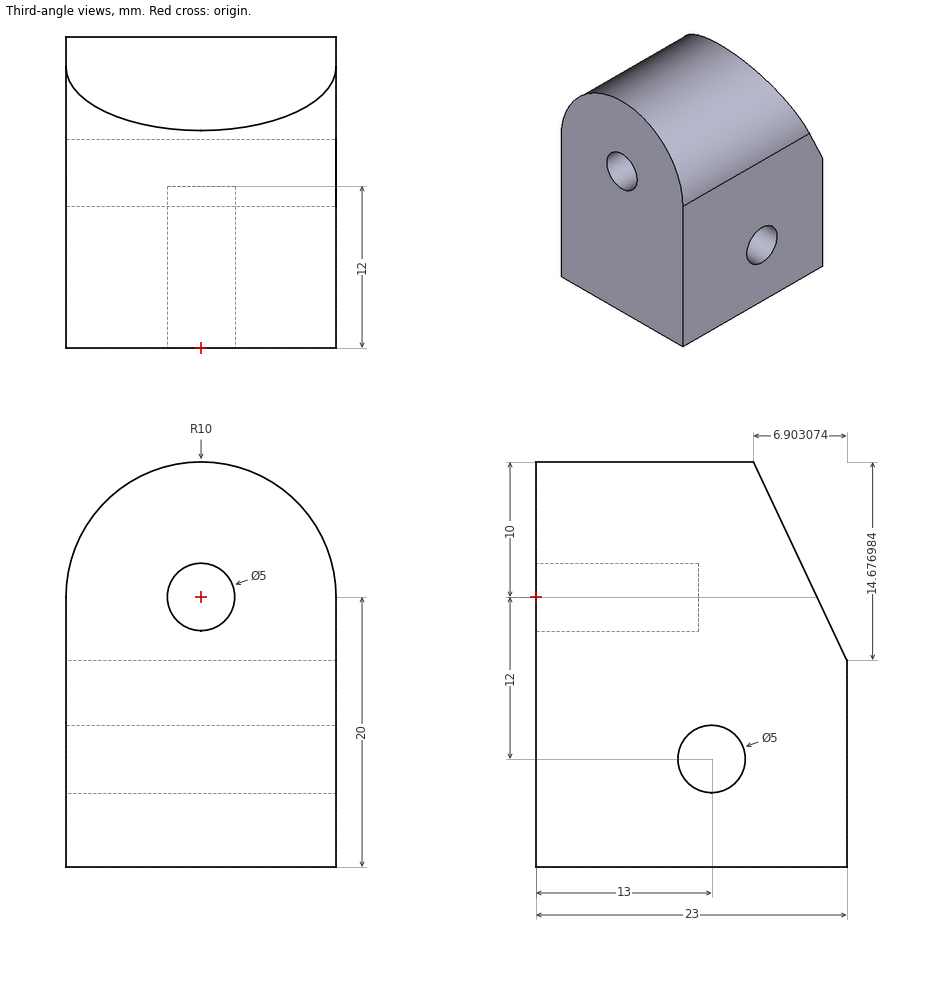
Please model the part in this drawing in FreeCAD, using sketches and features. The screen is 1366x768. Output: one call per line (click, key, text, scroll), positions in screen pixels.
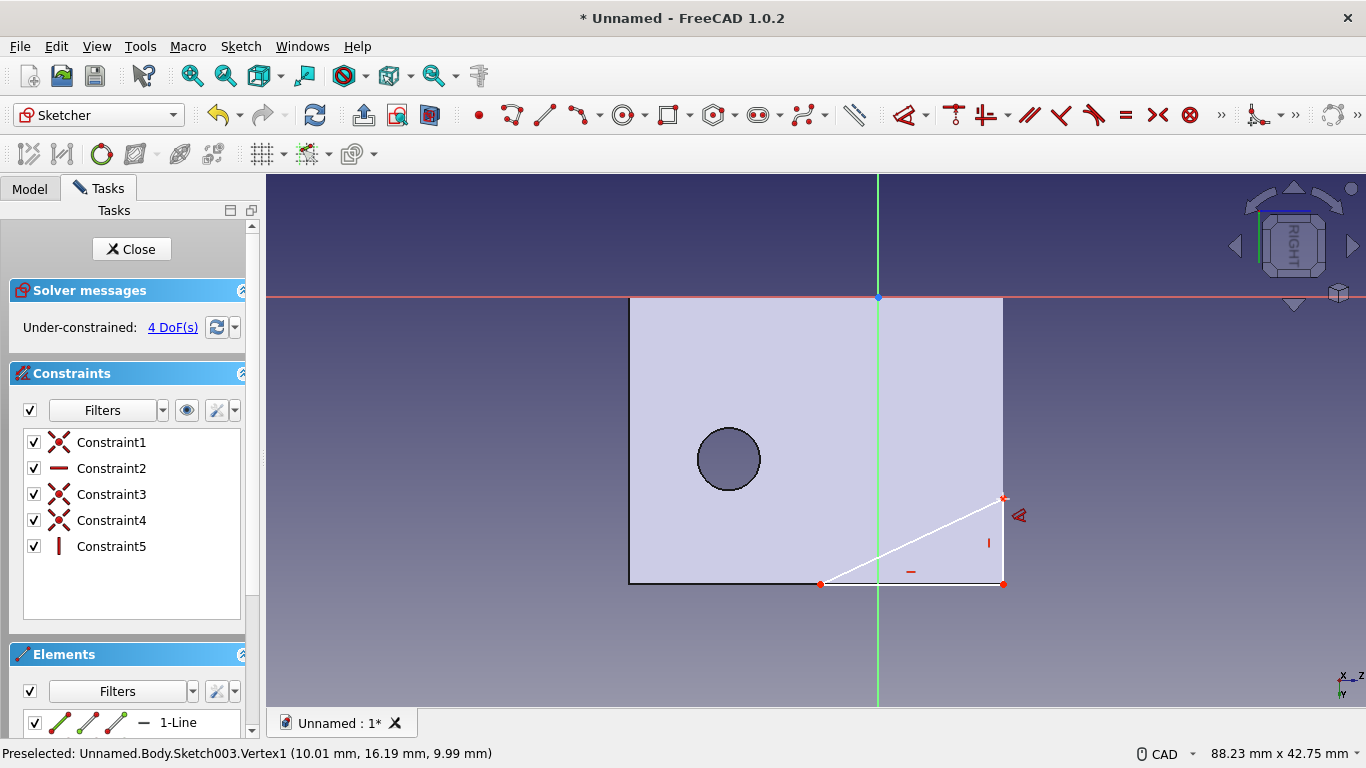
click(1003, 499)
click(941, 263)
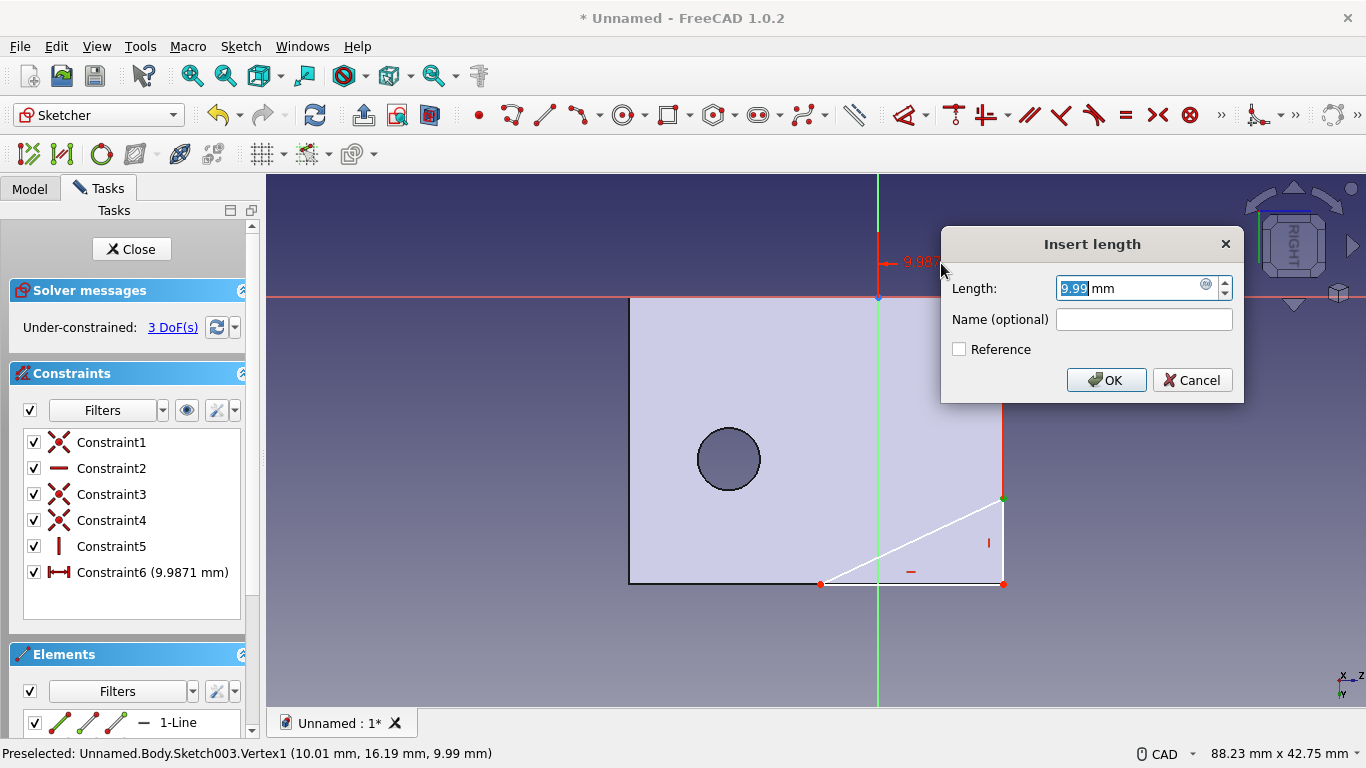
text(10)
key(Return)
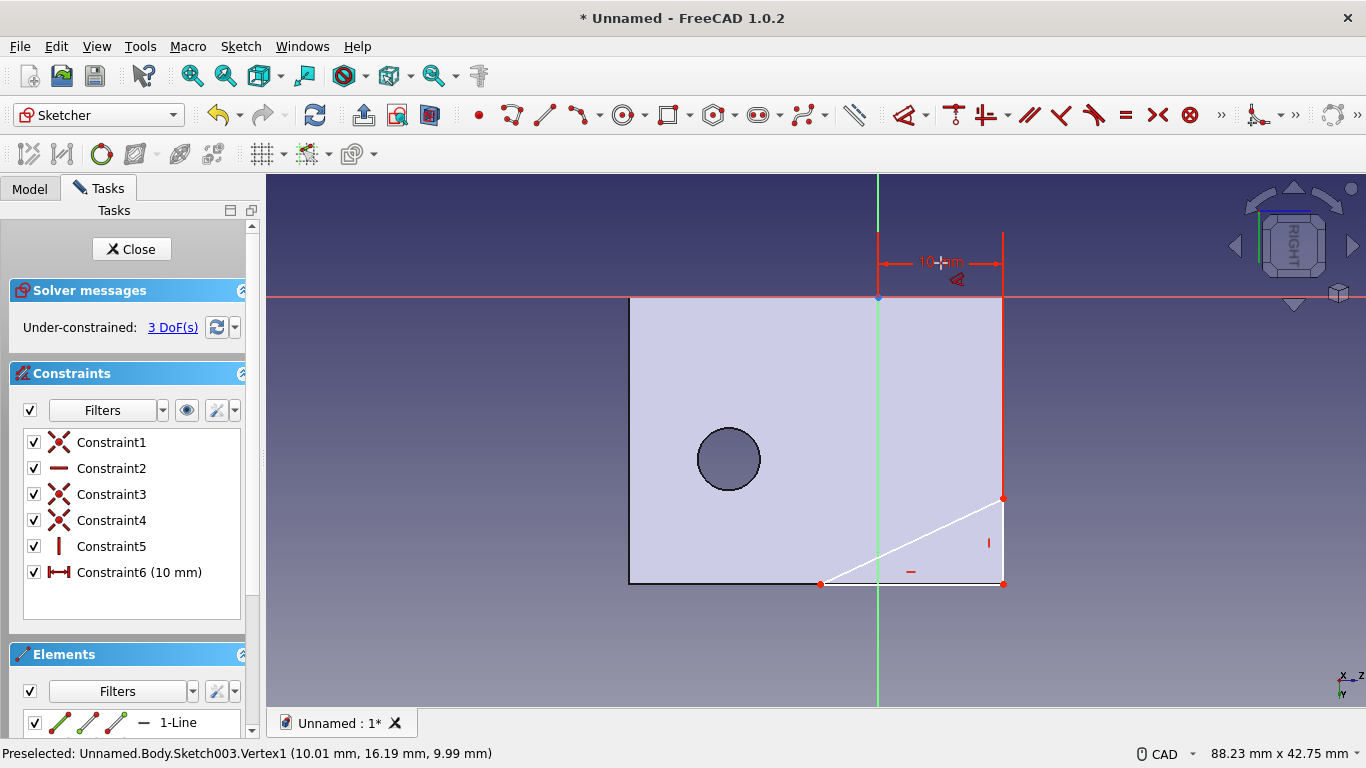
click(820, 585)
click(786, 441)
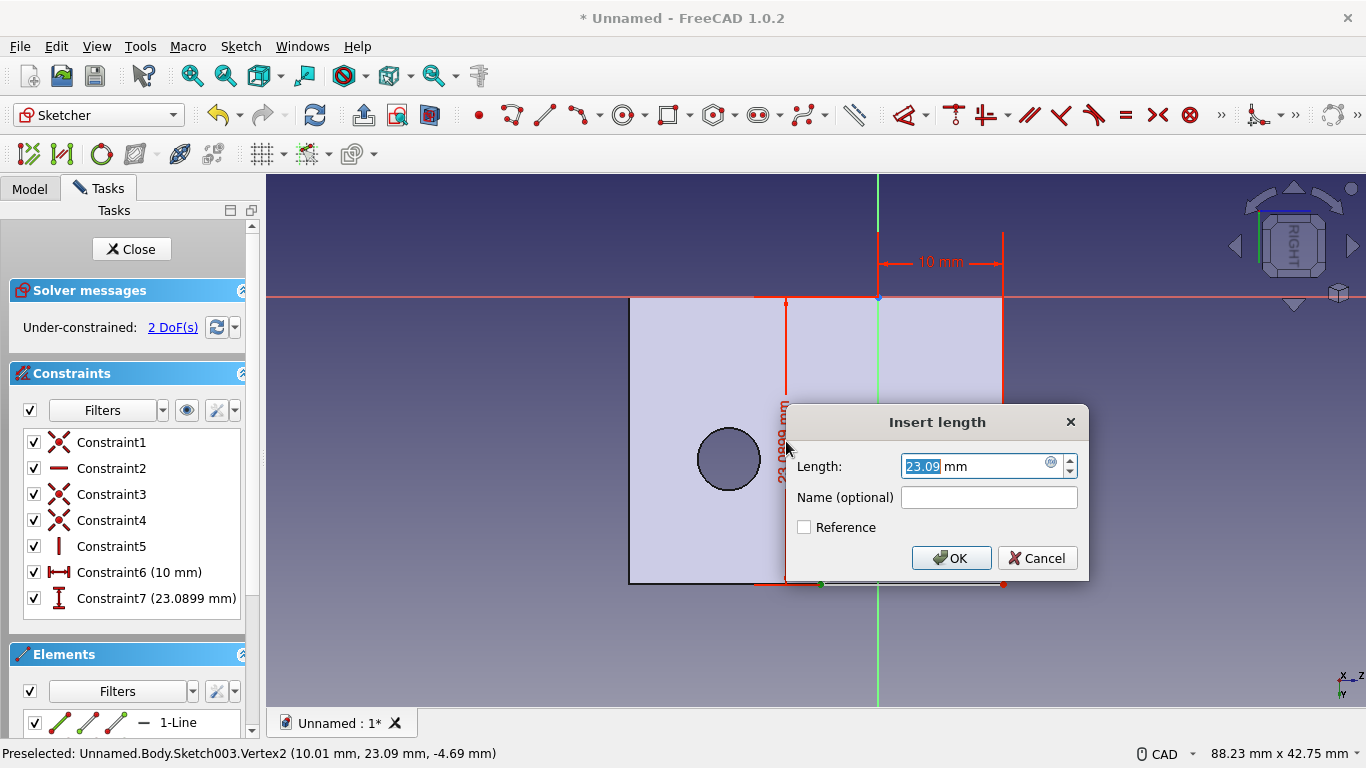
text(23)
key(Return)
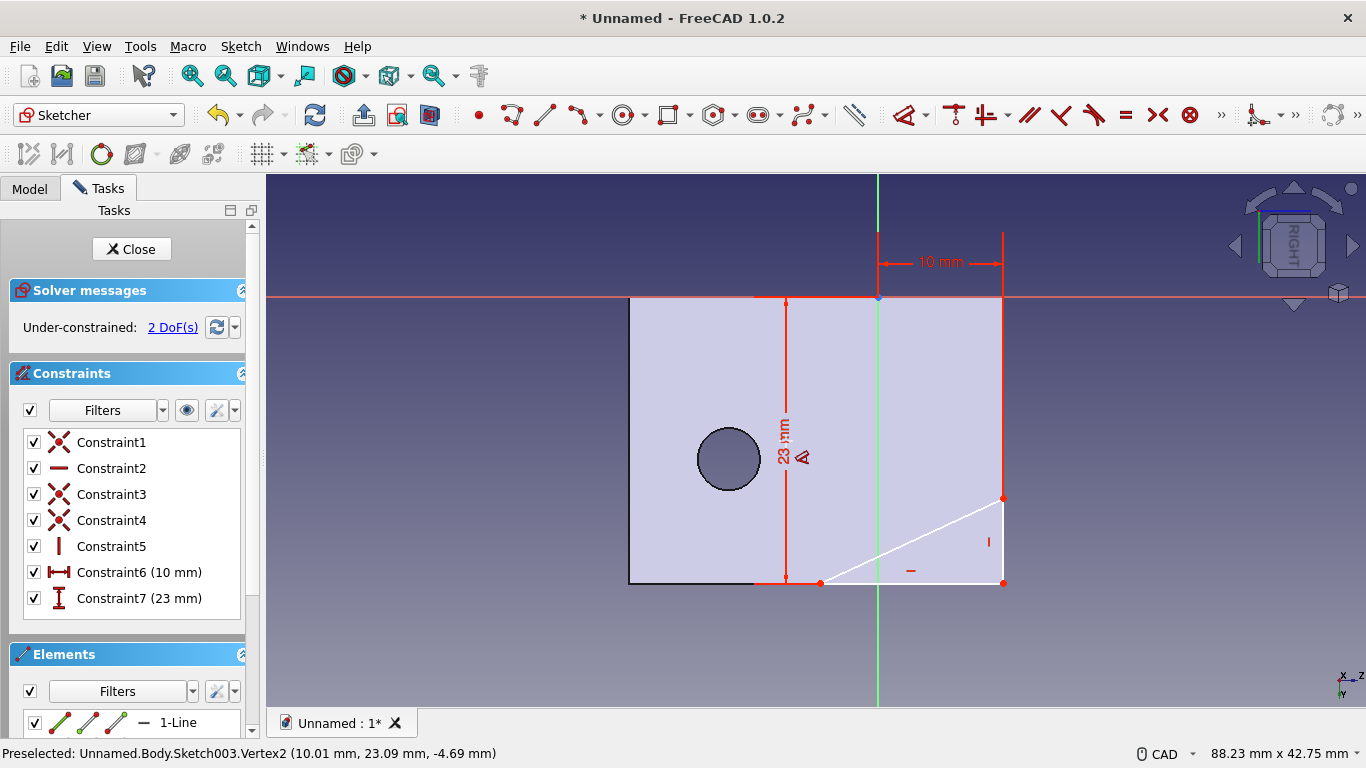
click(1003, 558)
click(1037, 541)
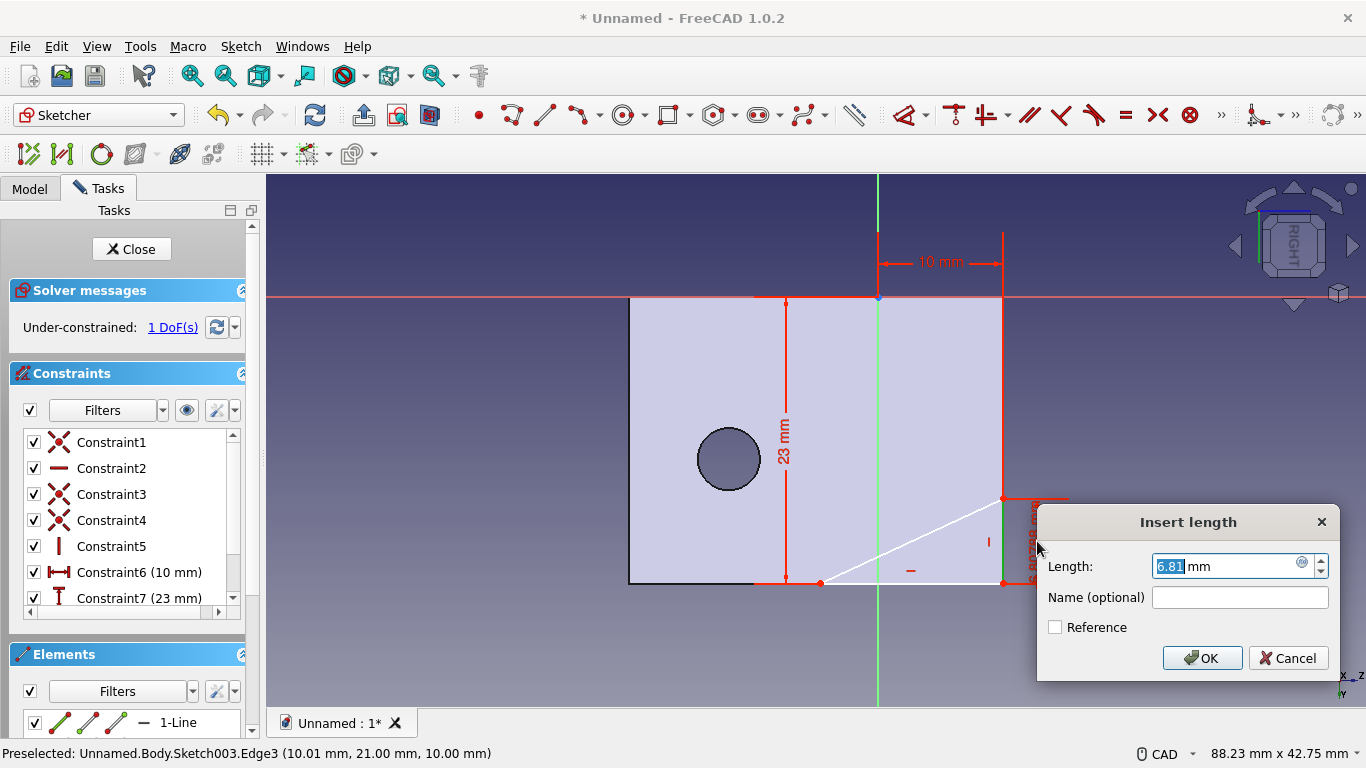
text(6.903074)
key(Return)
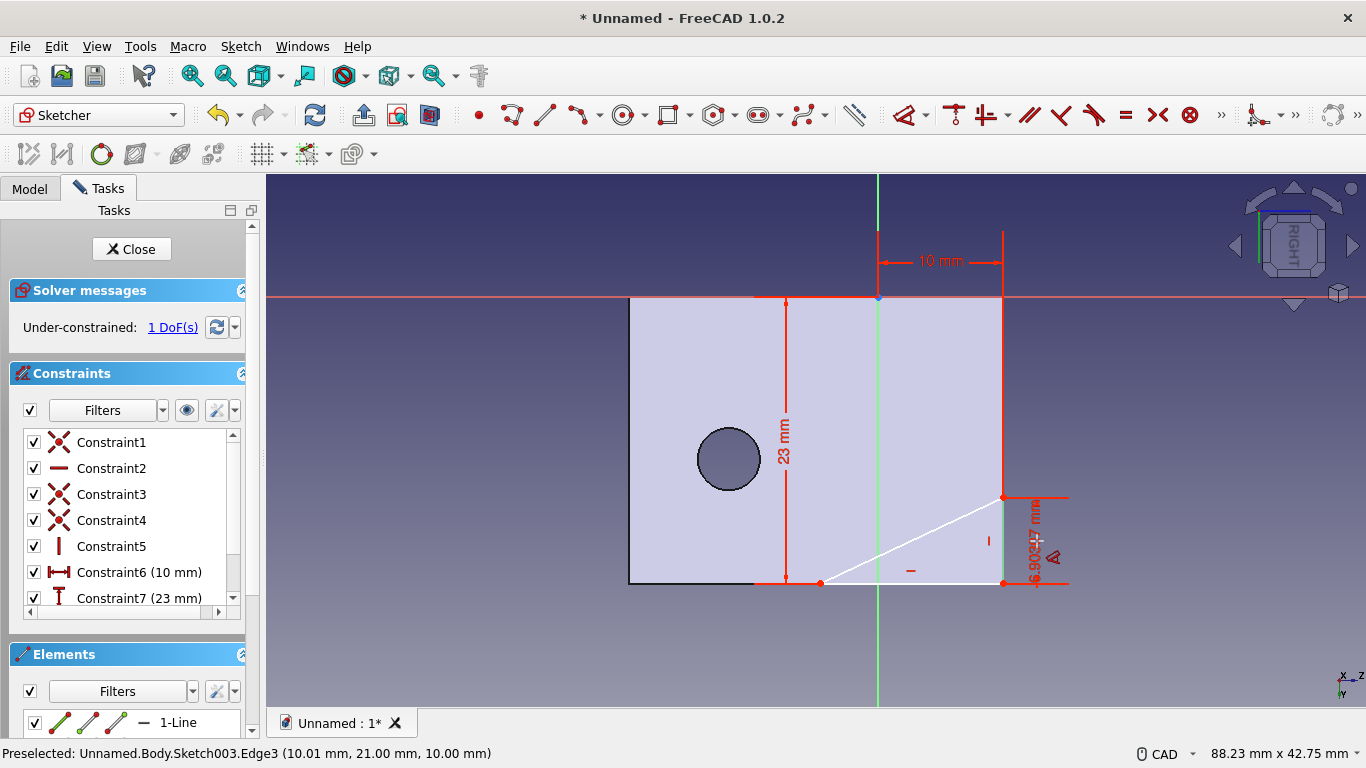
click(875, 584)
click(912, 618)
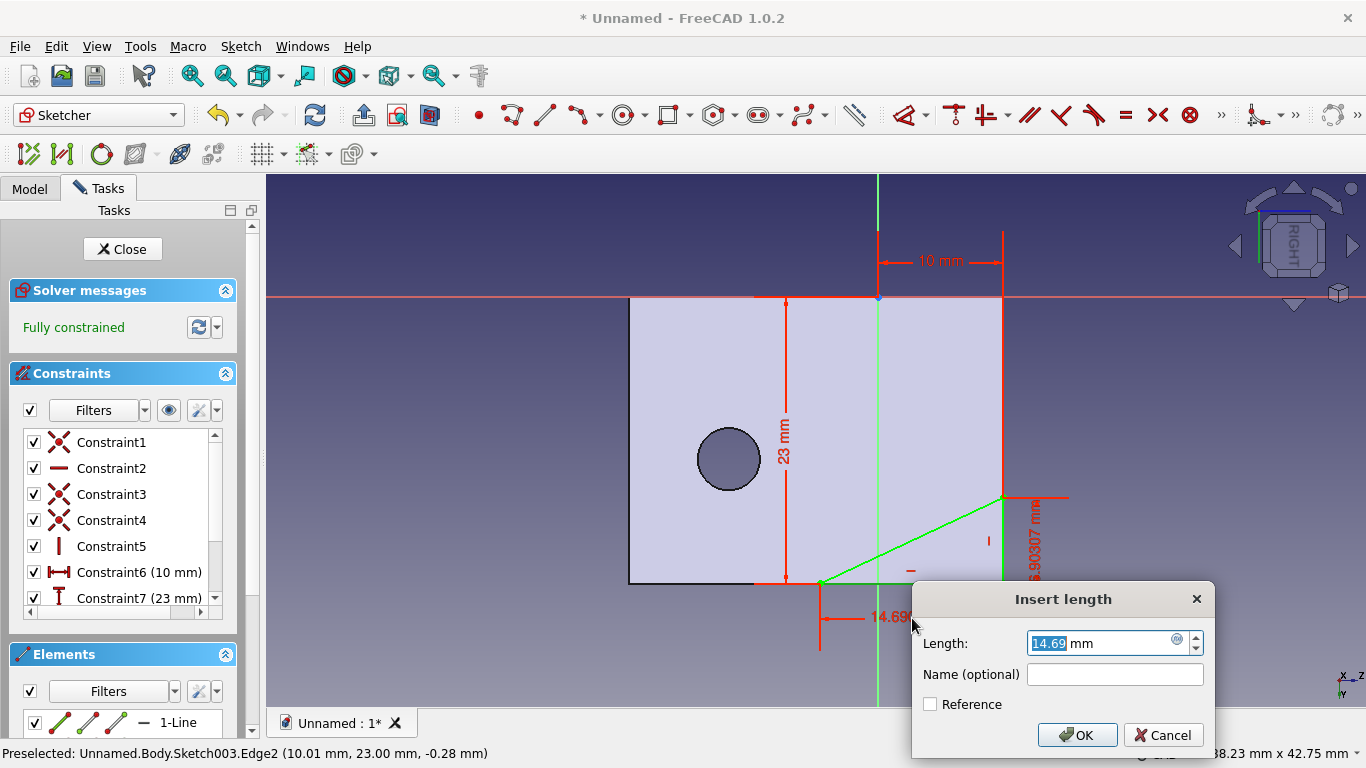
text(14.676984)
key(Return)
key(Escape)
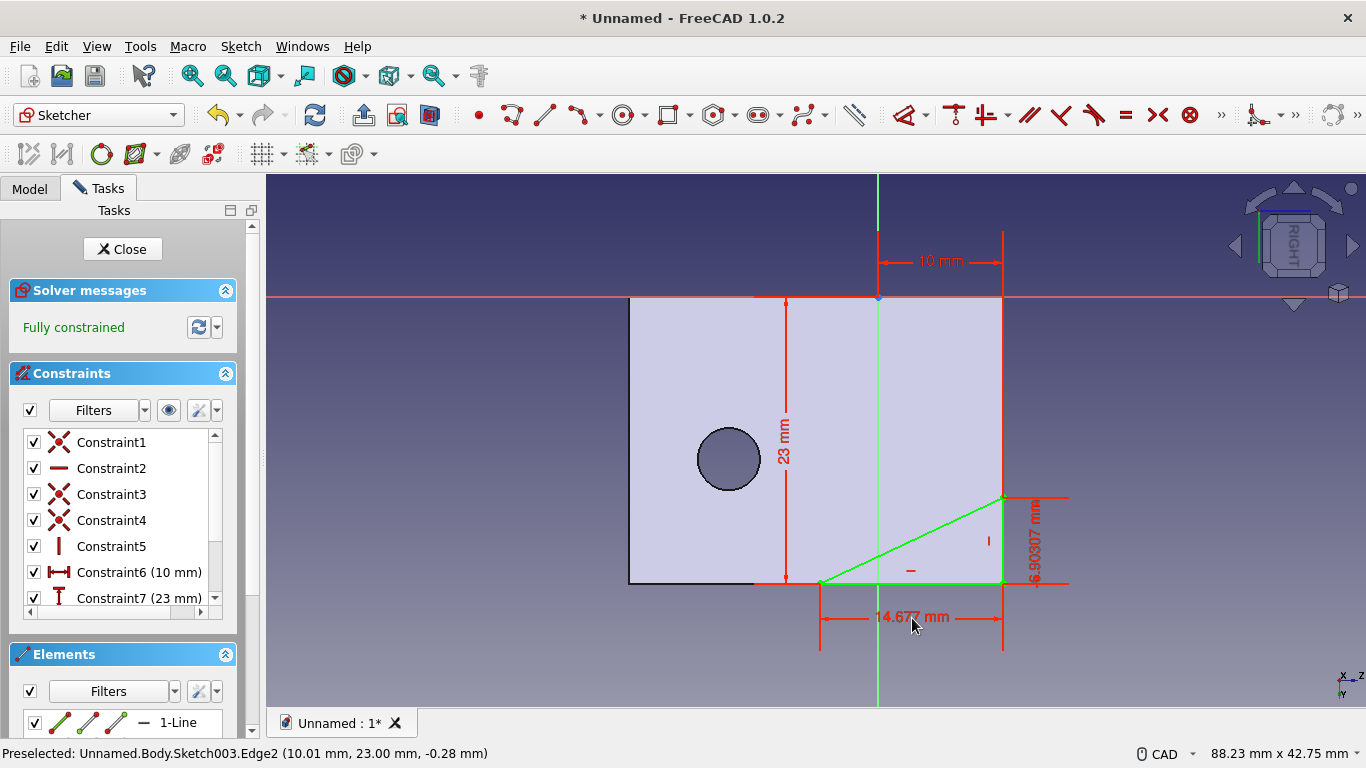
click(123, 249)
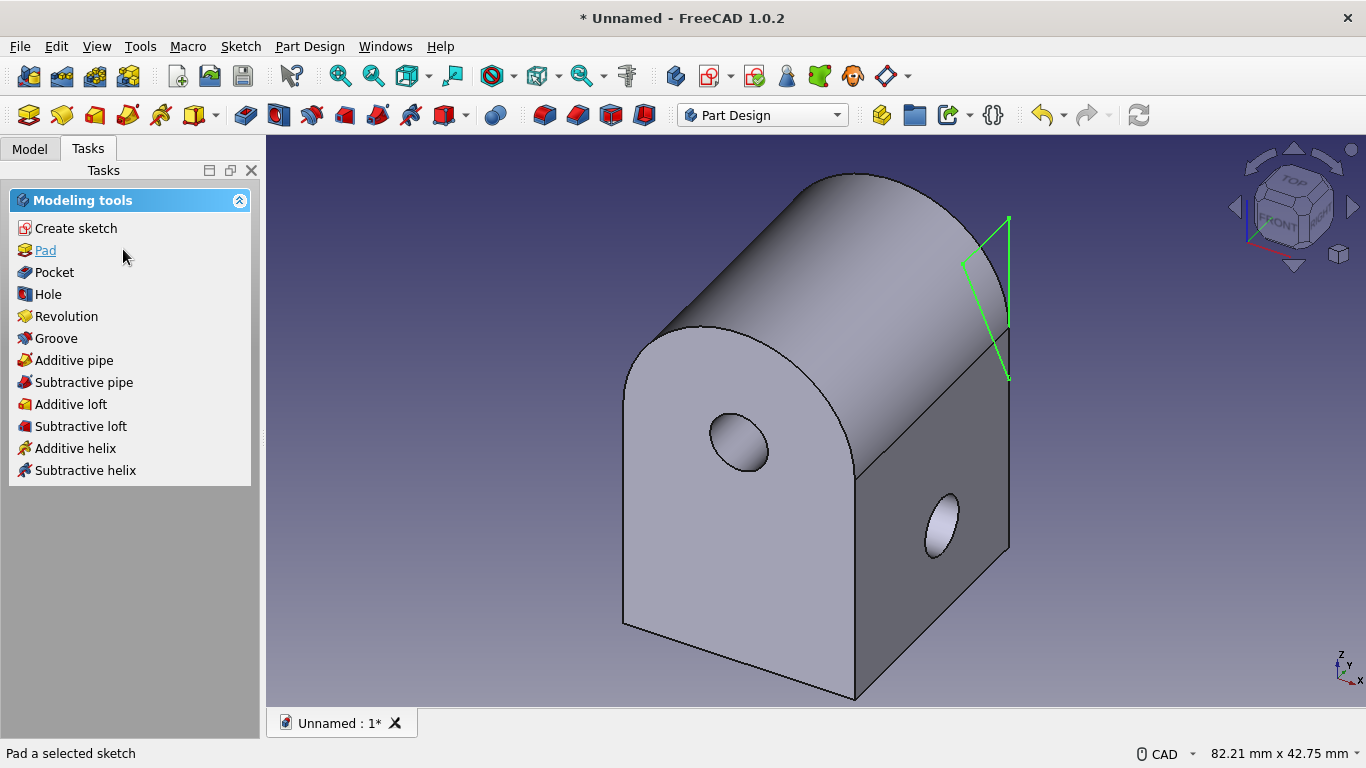
click(246, 116)